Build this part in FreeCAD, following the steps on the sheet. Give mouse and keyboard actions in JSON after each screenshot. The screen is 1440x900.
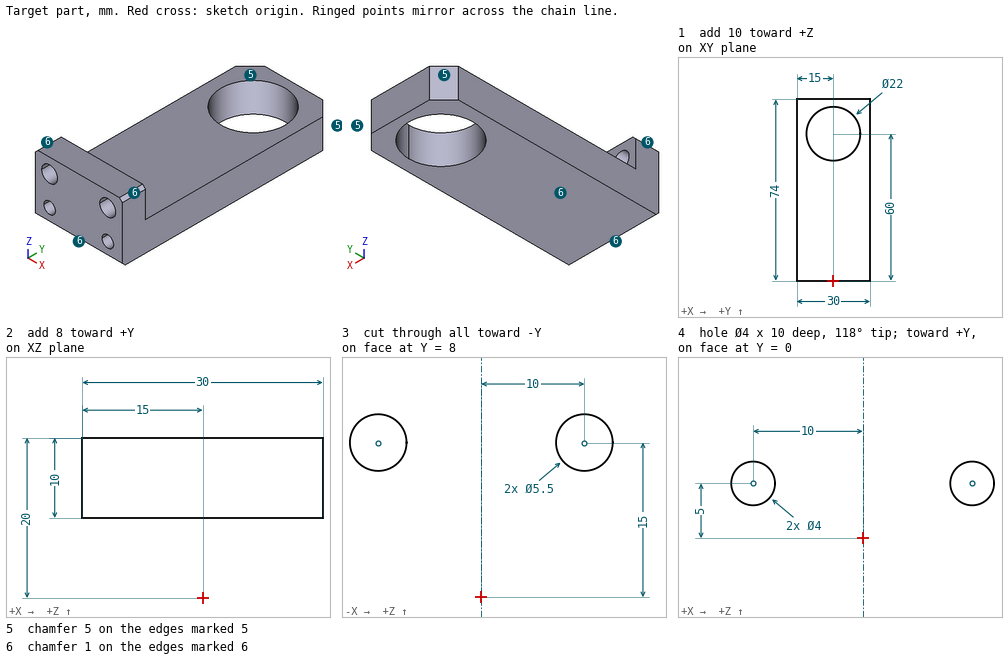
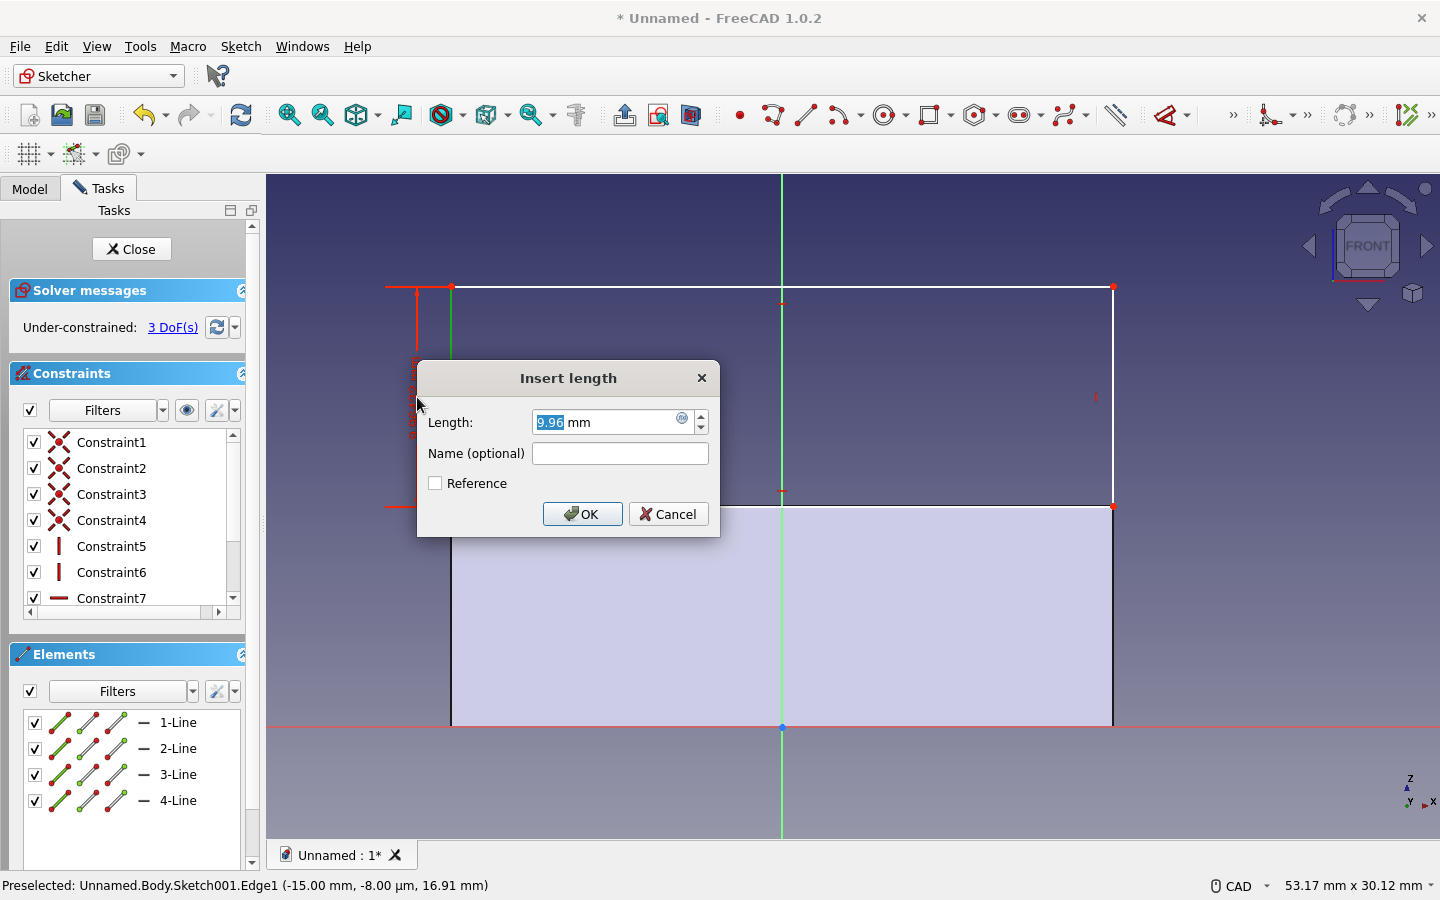
{"action": "type", "text": "10"}
{"action": "key", "text": "Return"}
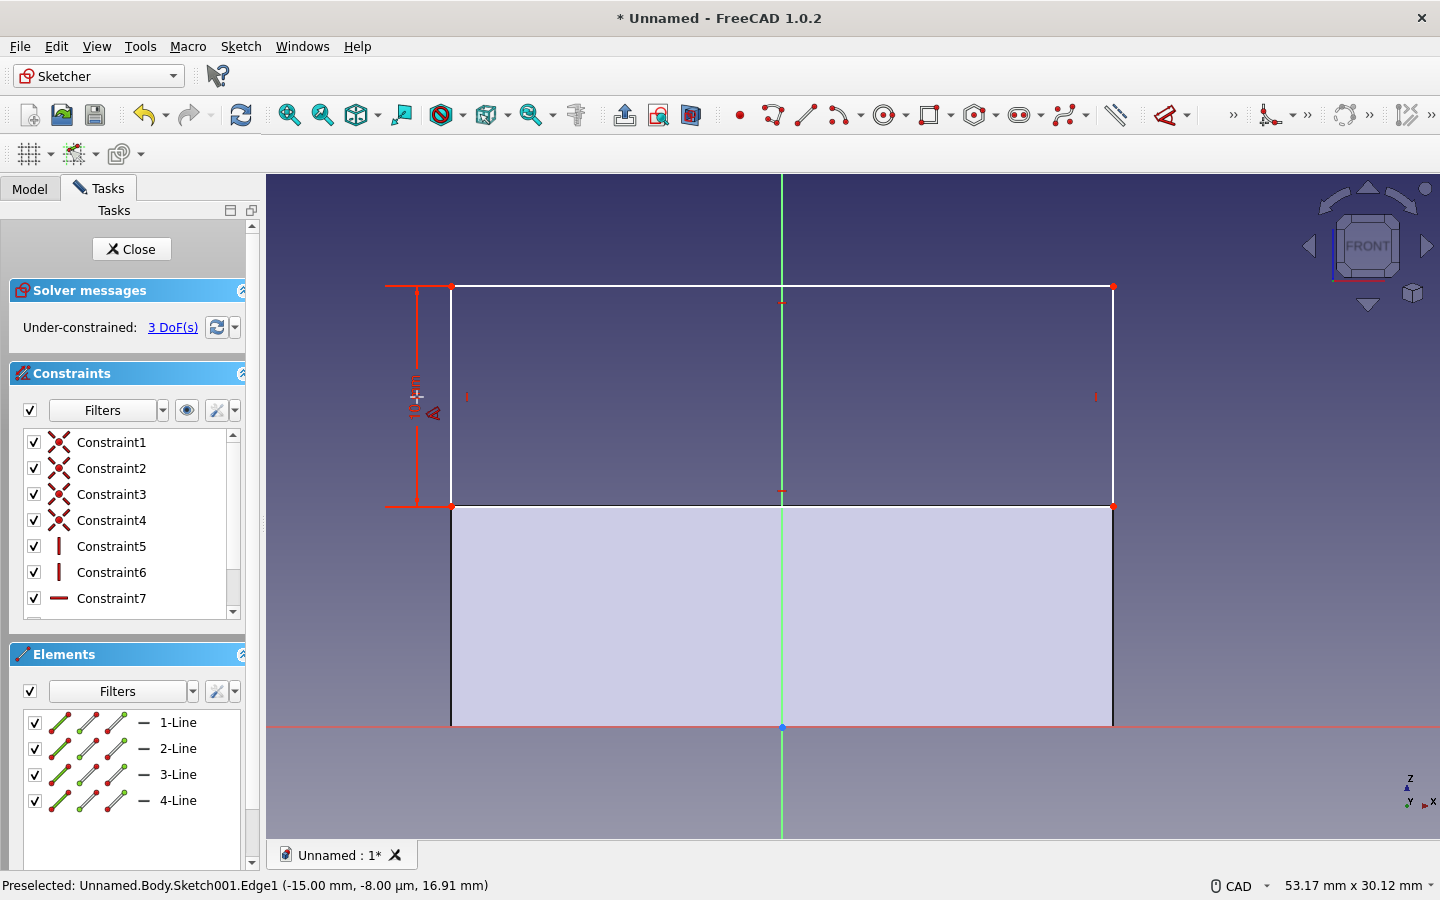
{"action": "left_click", "coordinate": [650, 507]}
{"action": "left_click", "coordinate": [630, 541]}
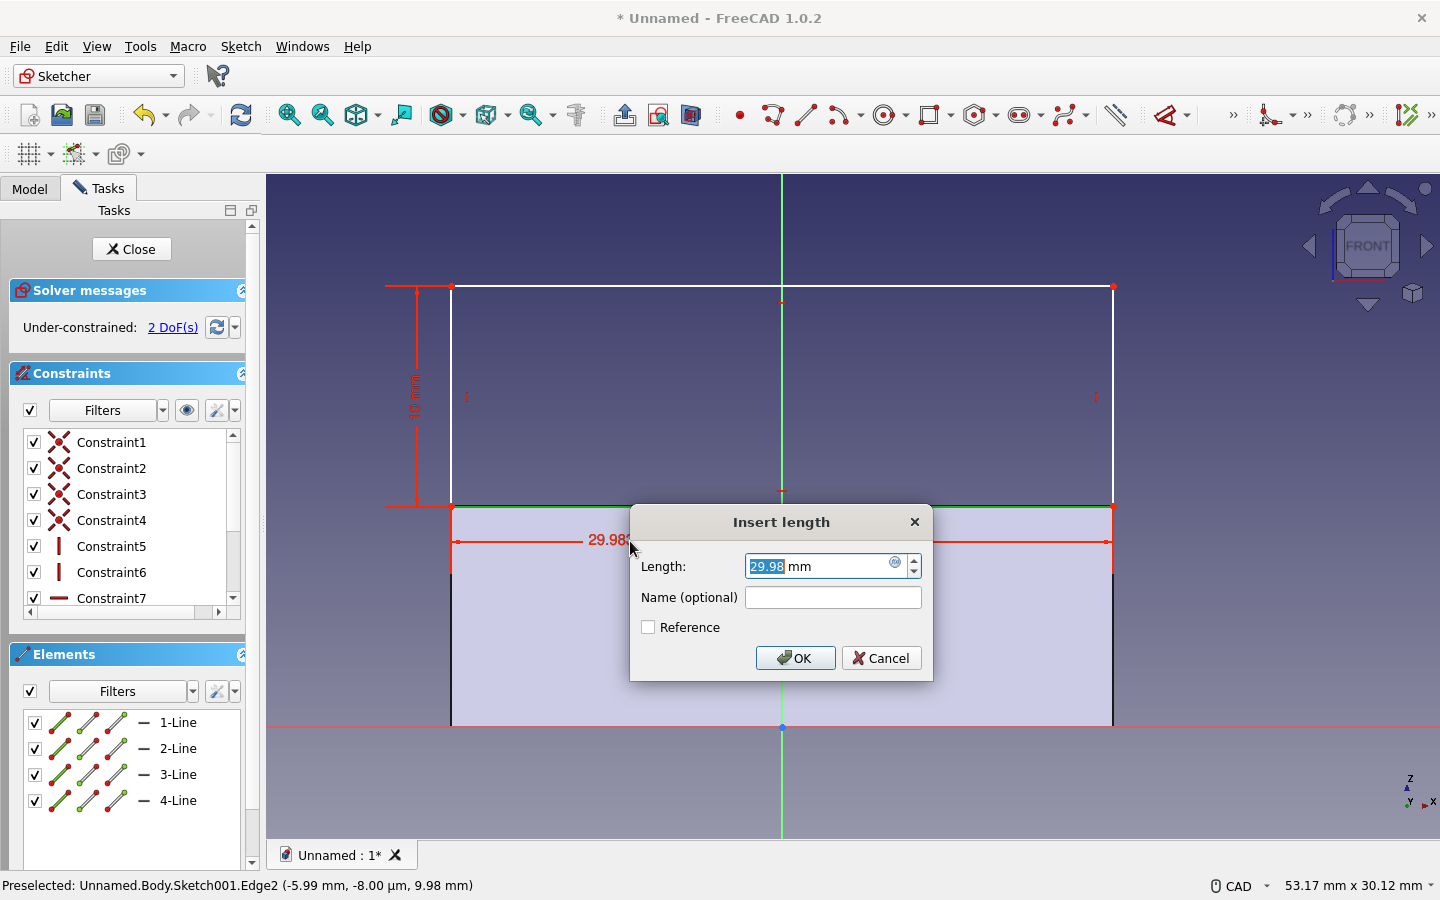
{"action": "type", "text": "30"}
{"action": "key", "text": "Return"}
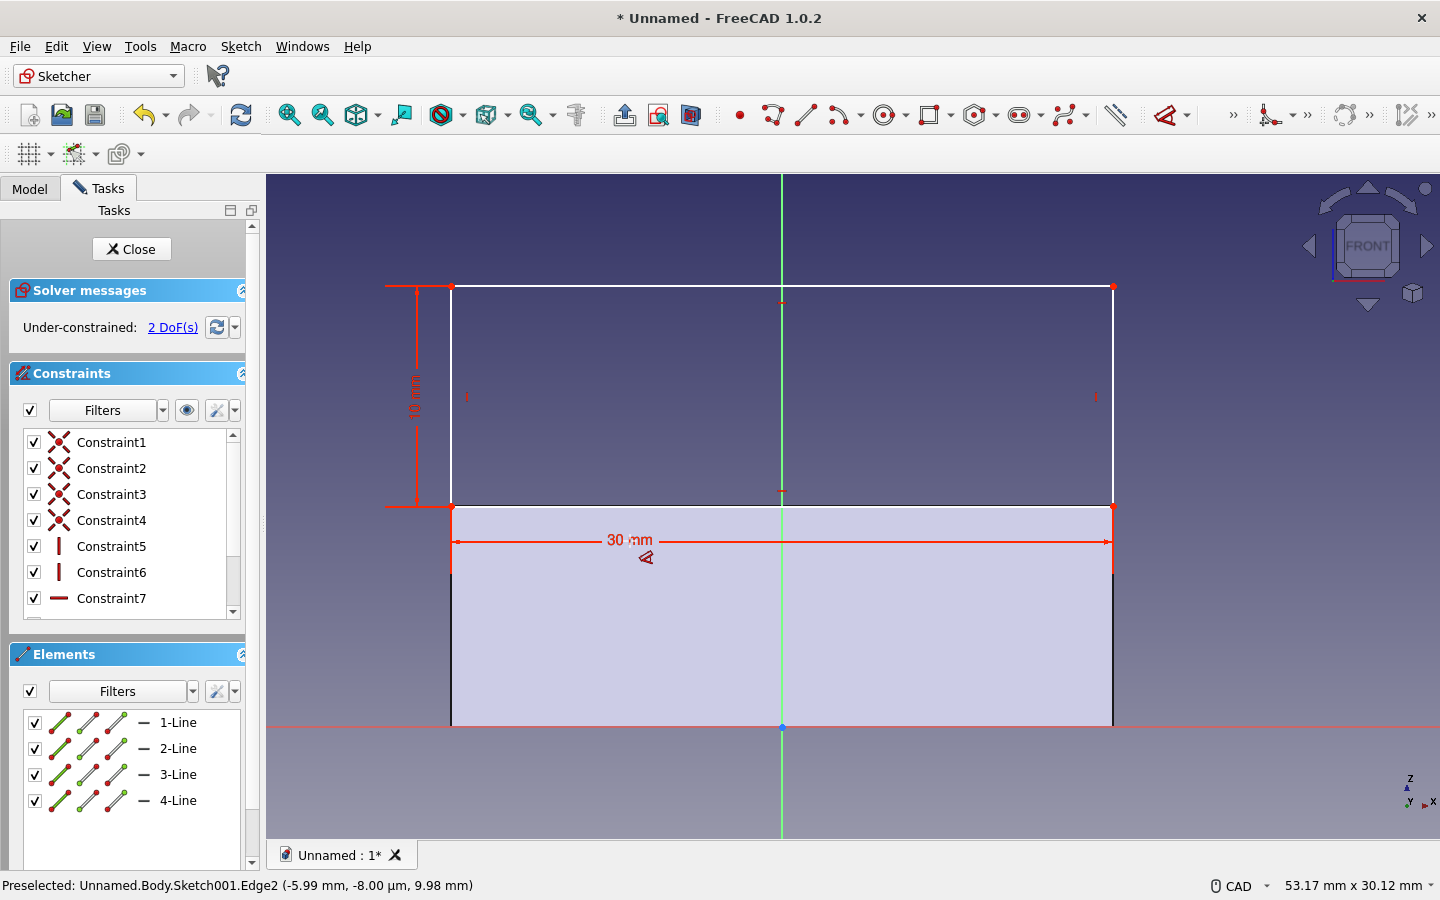
{"action": "left_click", "coordinate": [451, 286]}
{"action": "left_click", "coordinate": [617, 761]}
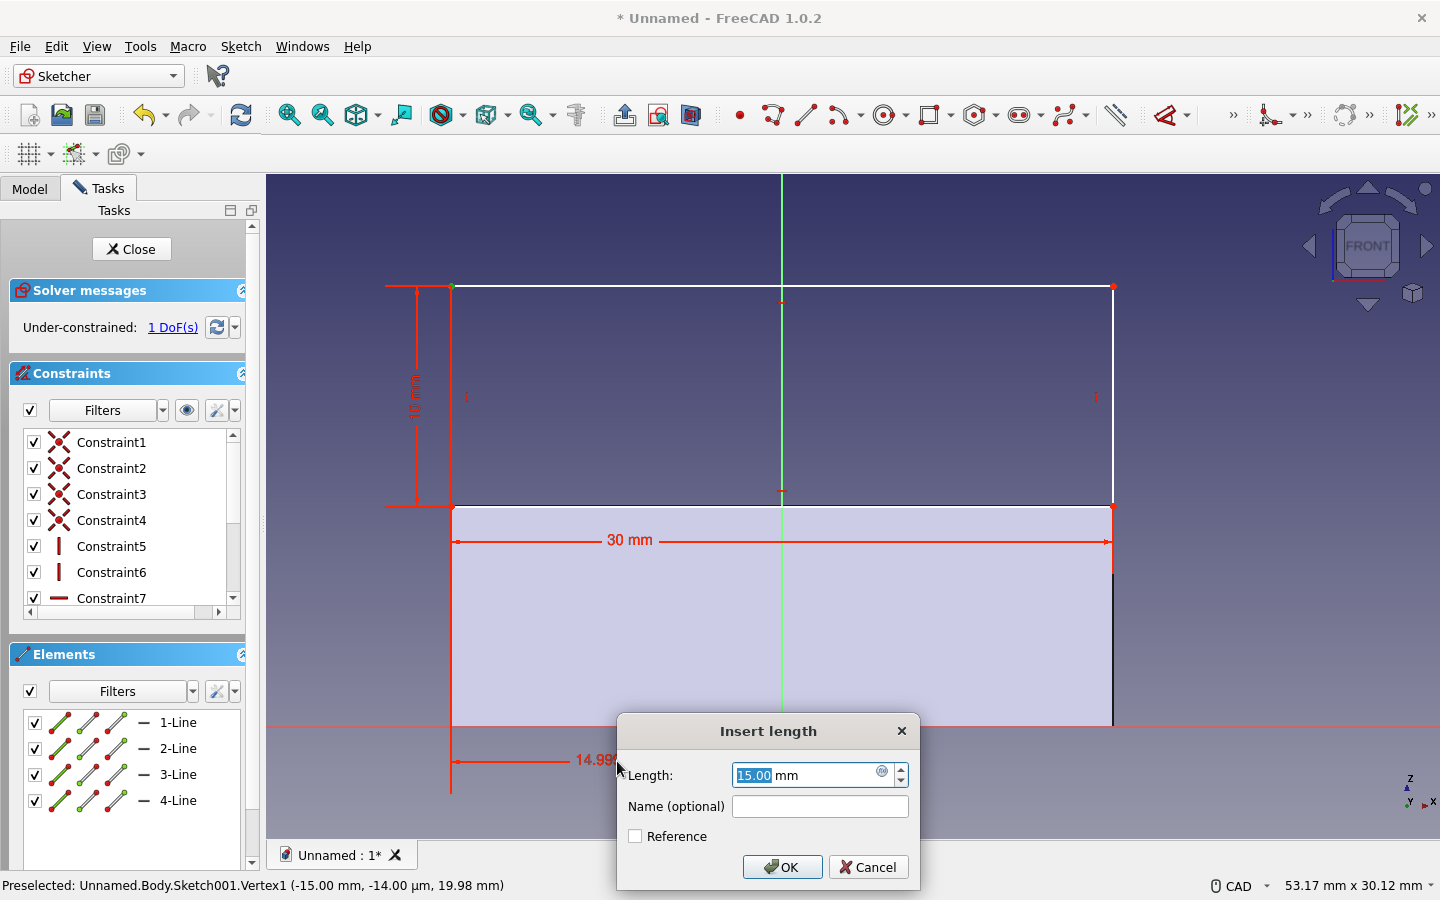
{"action": "type", "text": "15"}
{"action": "key", "text": "Return"}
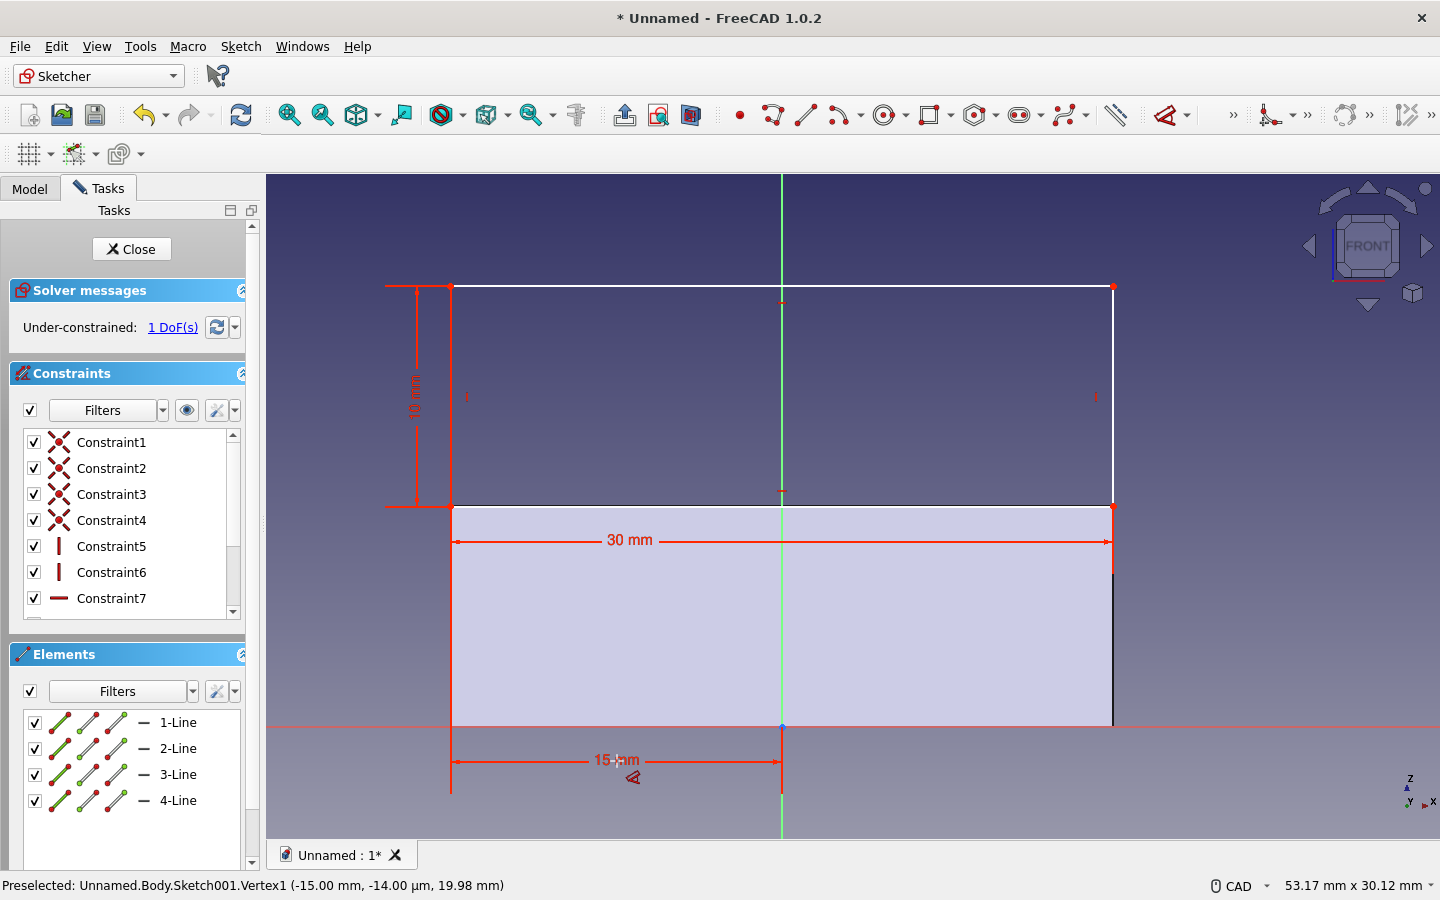
{"action": "left_click", "coordinate": [451, 286]}
{"action": "left_click", "coordinate": [417, 507]}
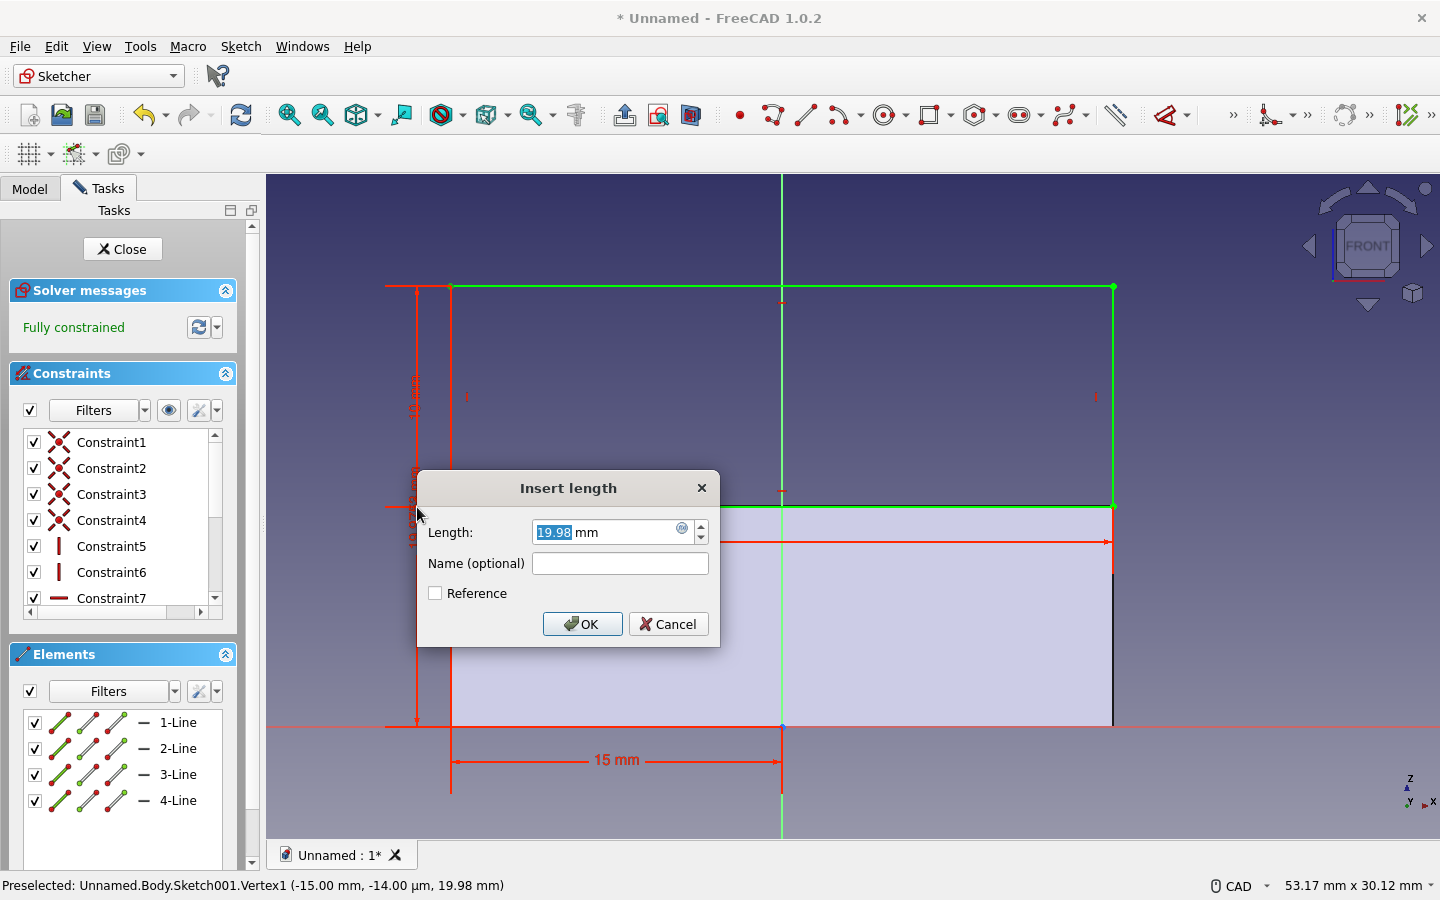
{"action": "type", "text": "20"}
{"action": "key", "text": "Return"}
{"action": "key", "text": "Escape"}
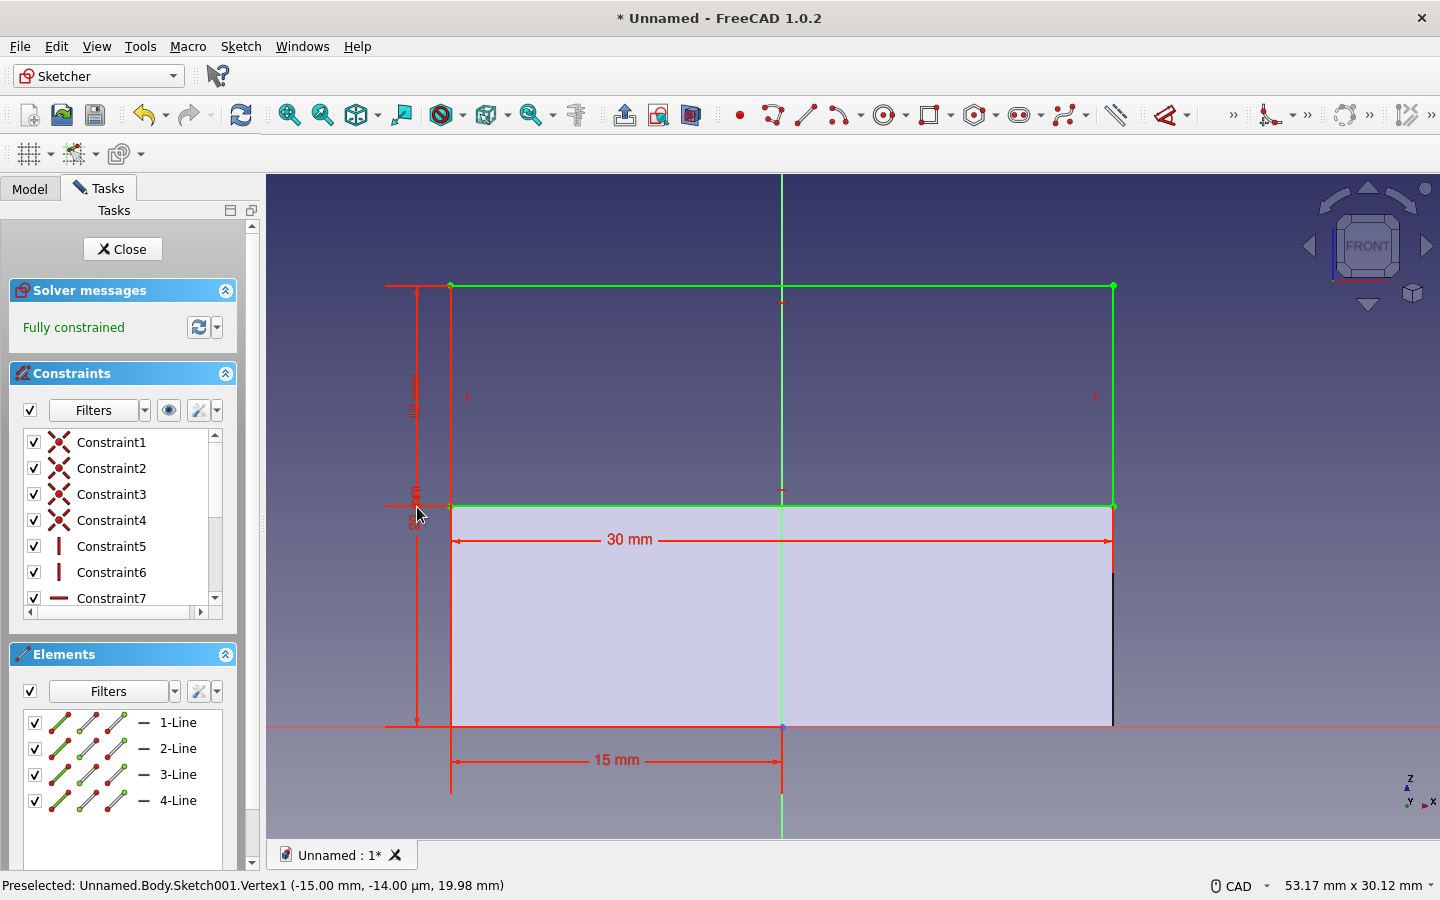
{"action": "left_click", "coordinate": [123, 249]}